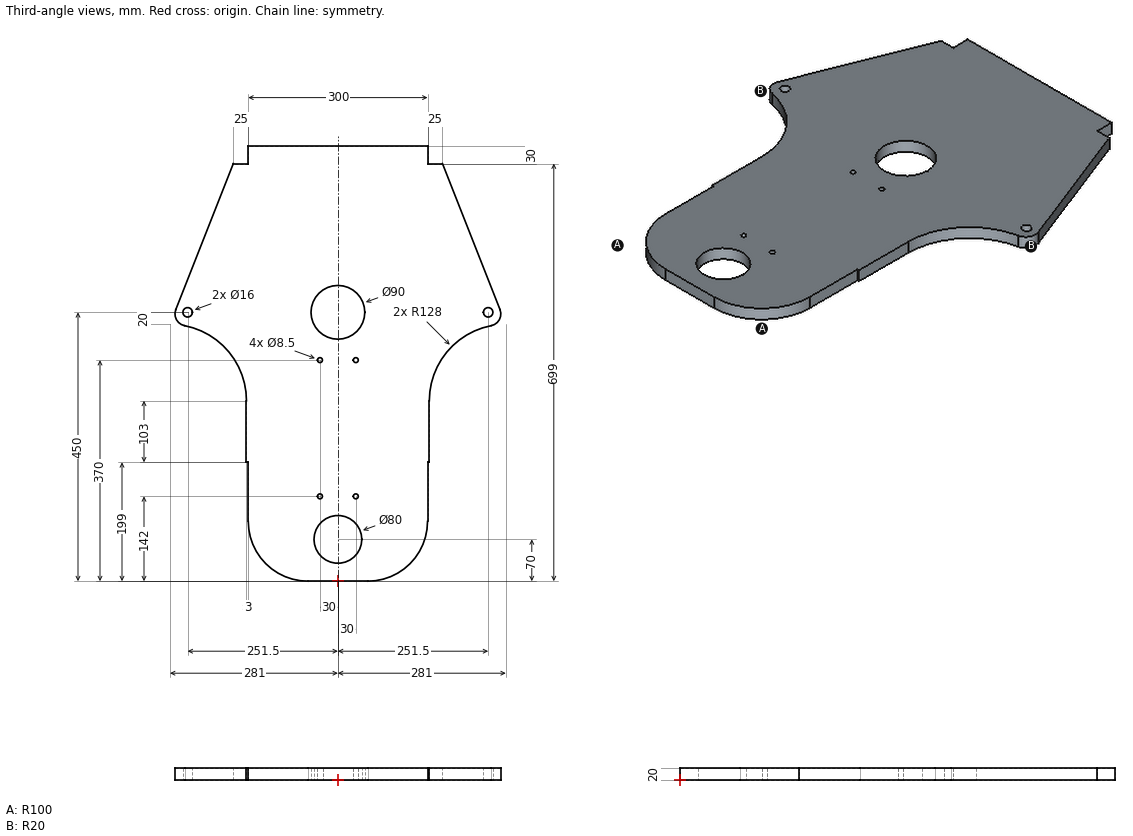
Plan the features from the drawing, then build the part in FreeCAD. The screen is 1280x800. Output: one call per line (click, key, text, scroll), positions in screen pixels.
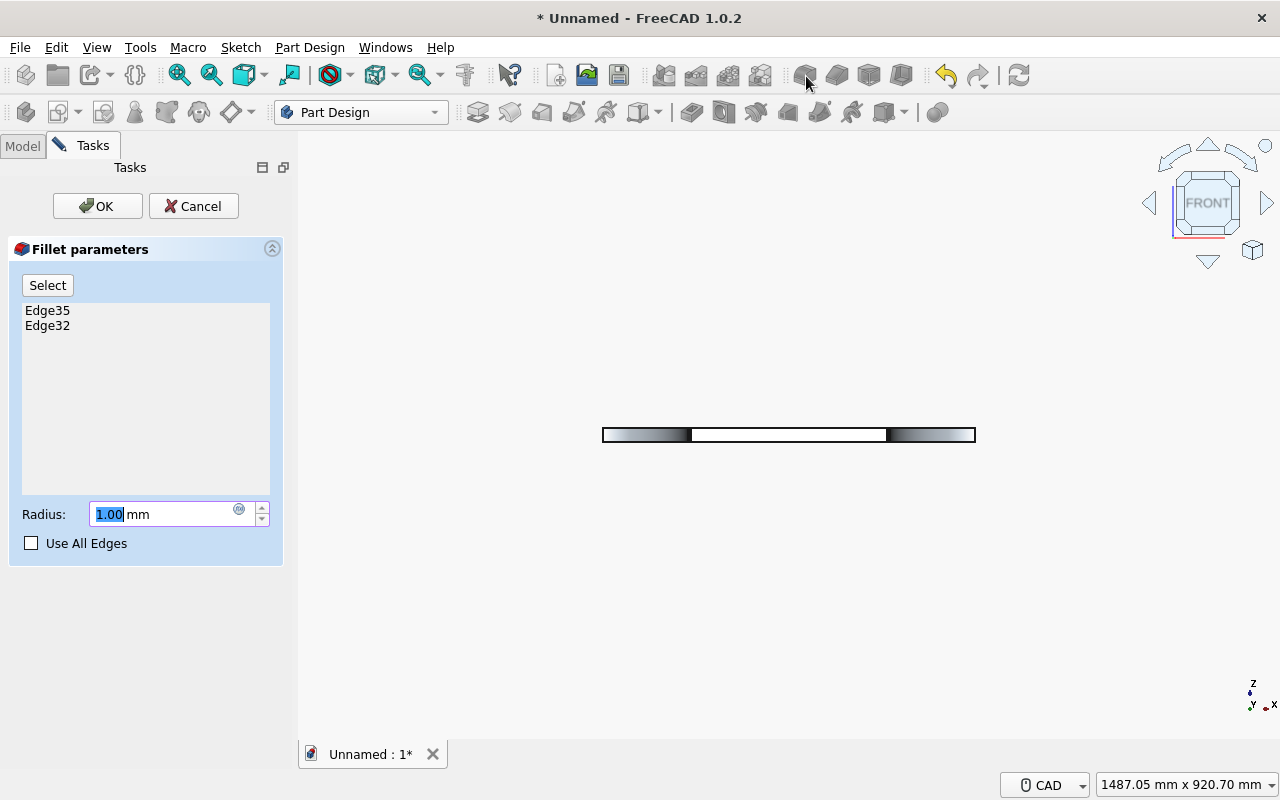
text(100)
key(Tab)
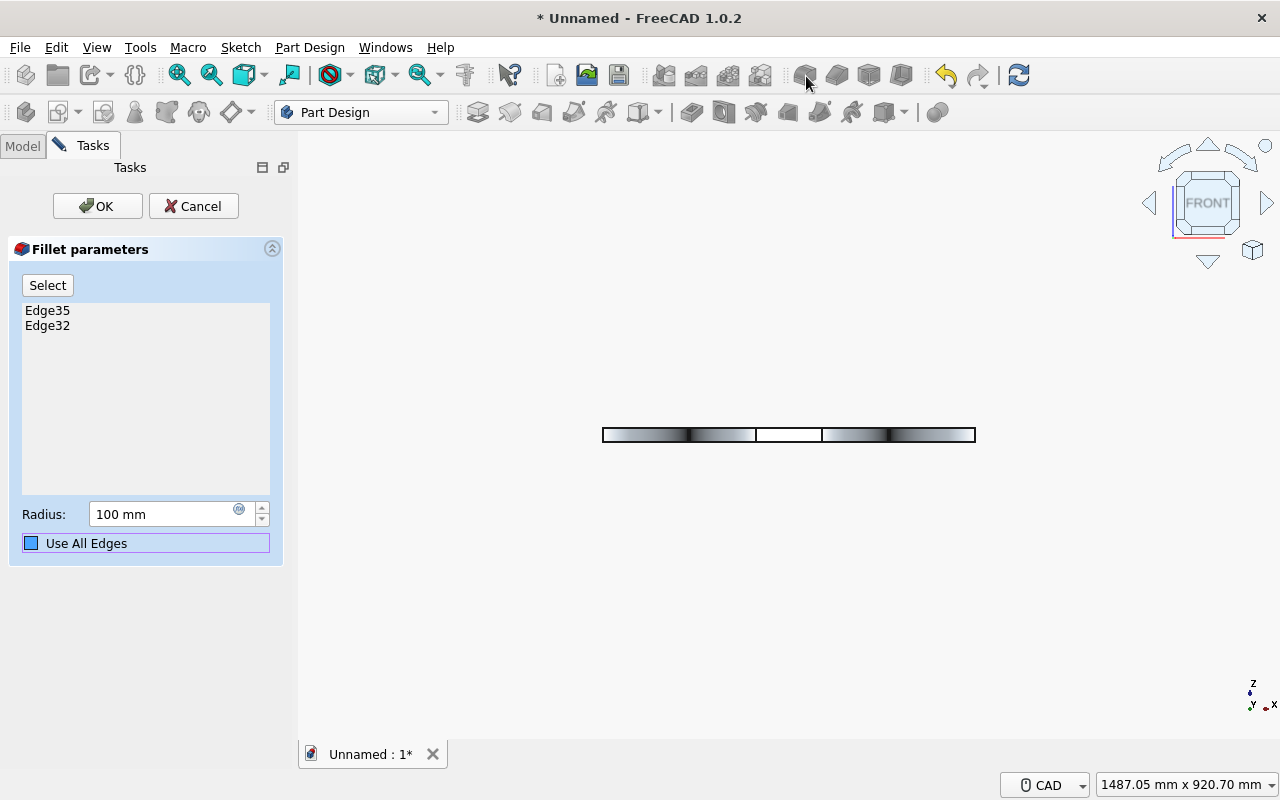
click(98, 206)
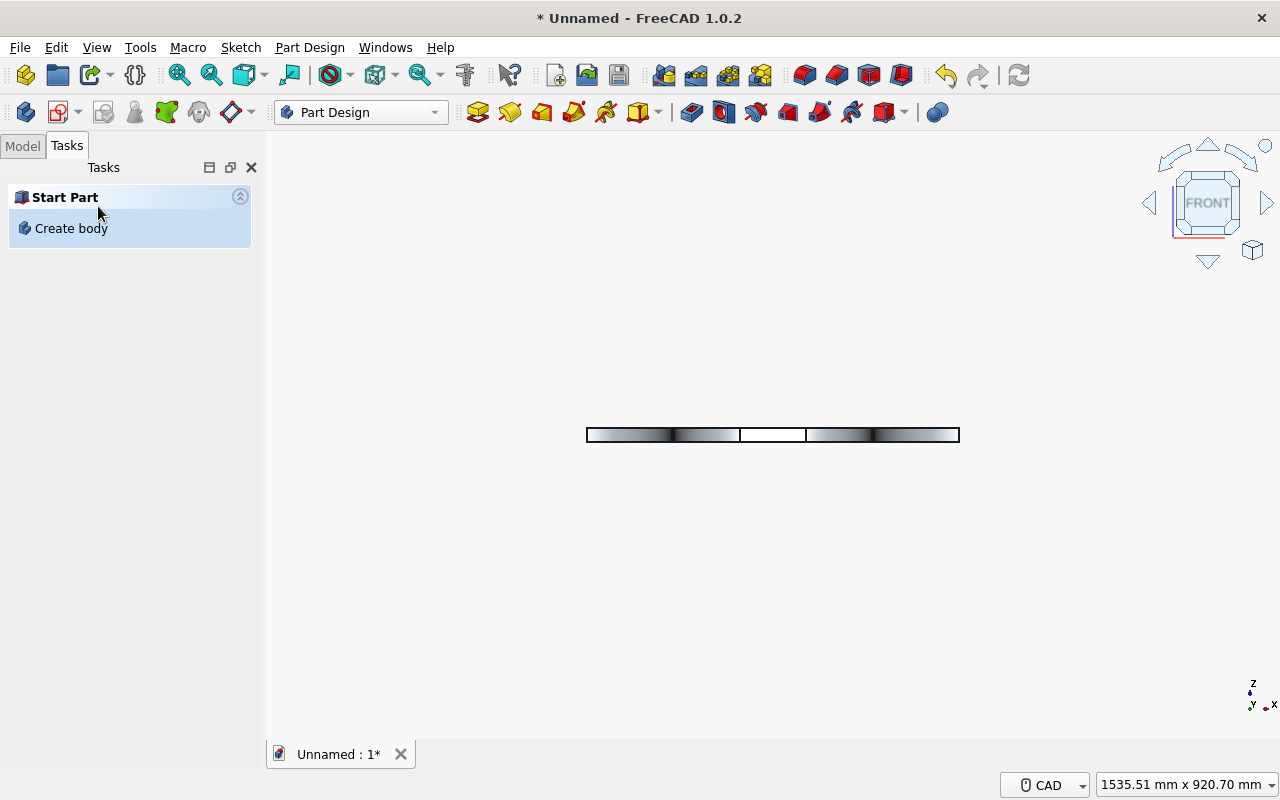
click(180, 76)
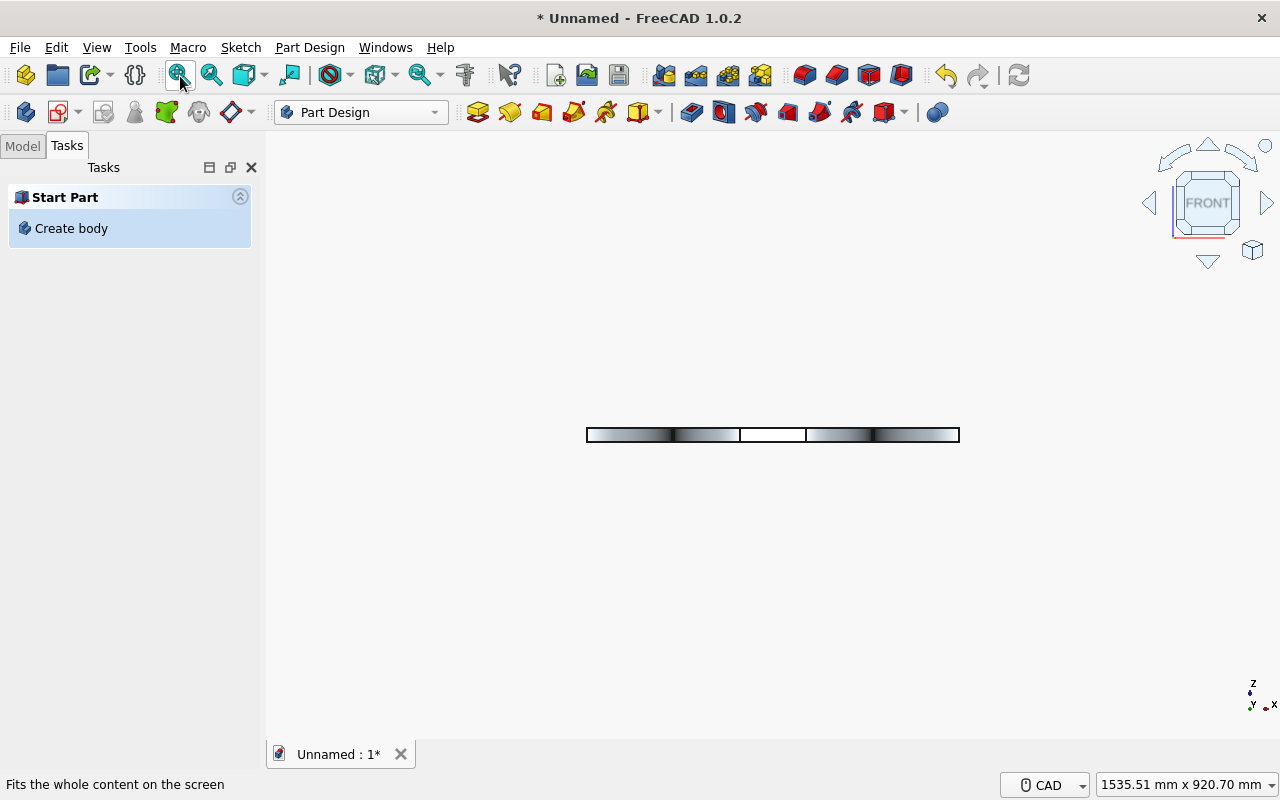
scroll(587, 434, up, 6)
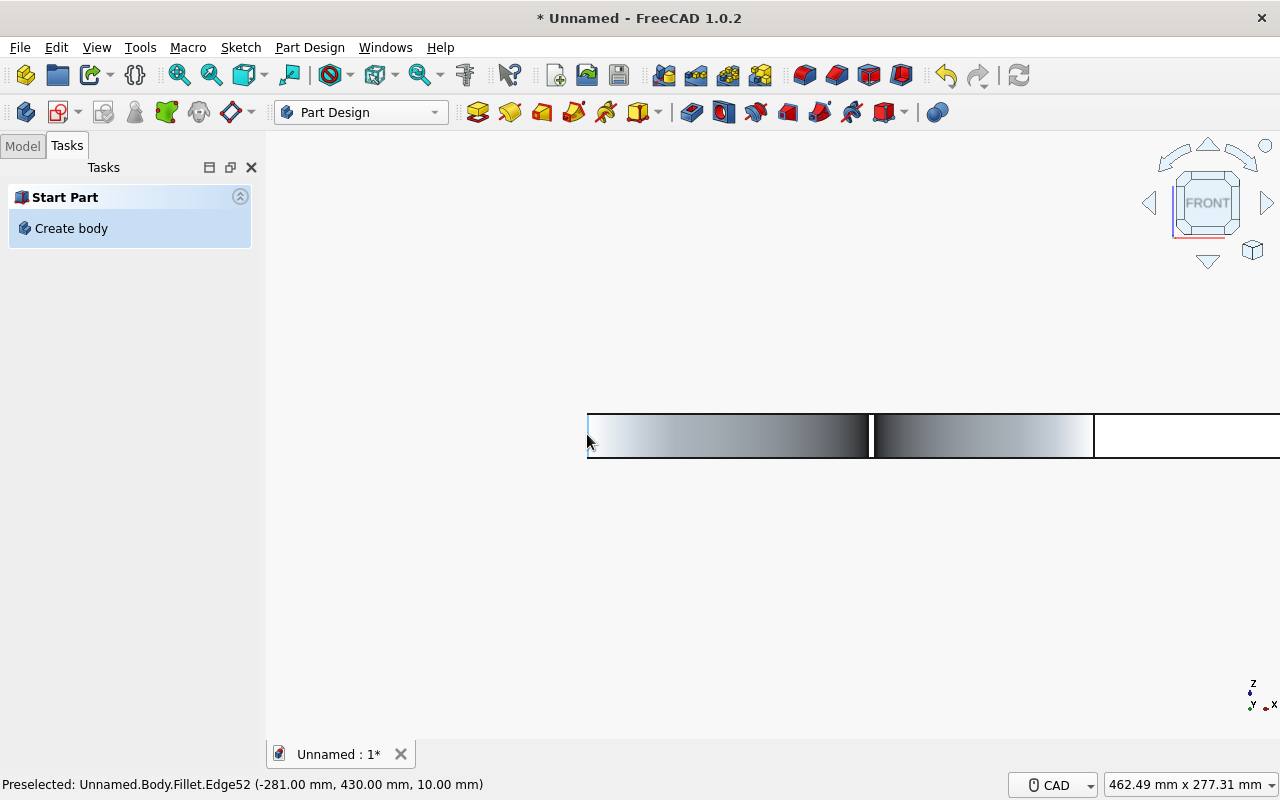
click(180, 76)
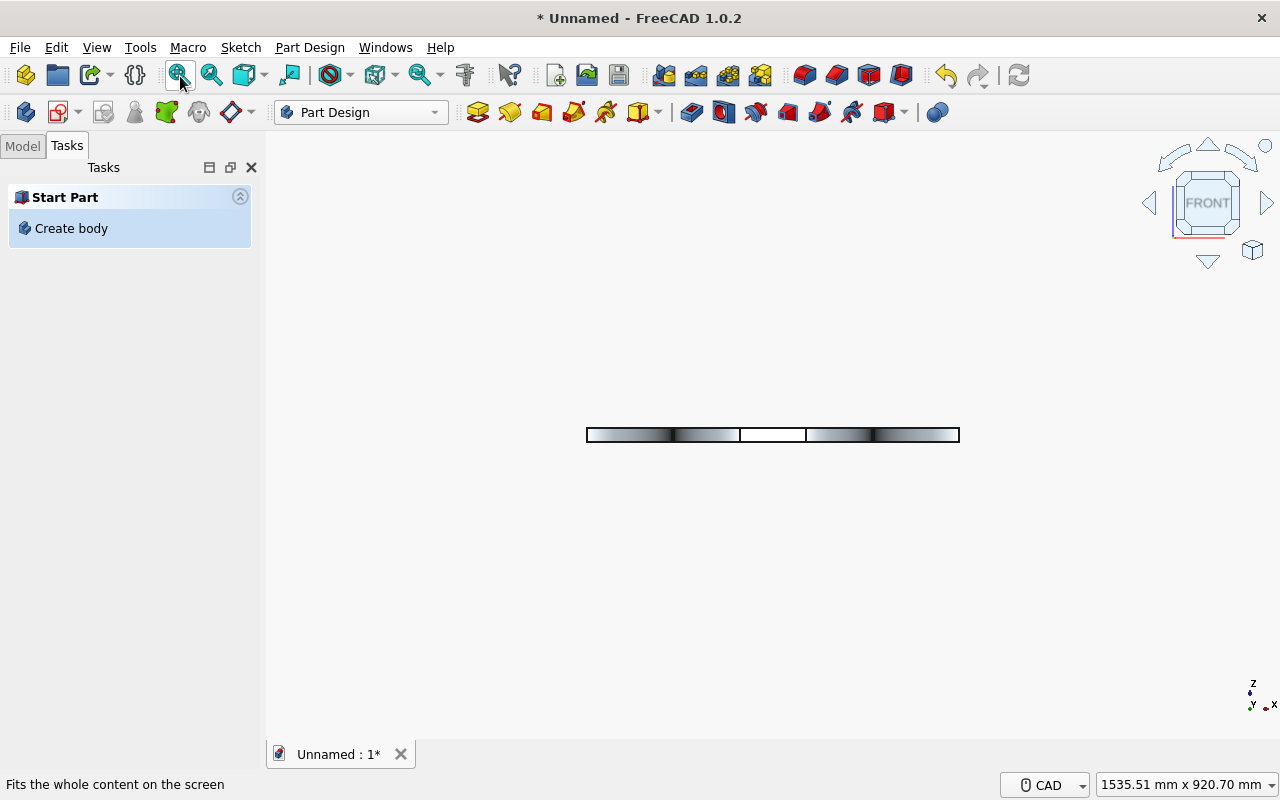
key(0)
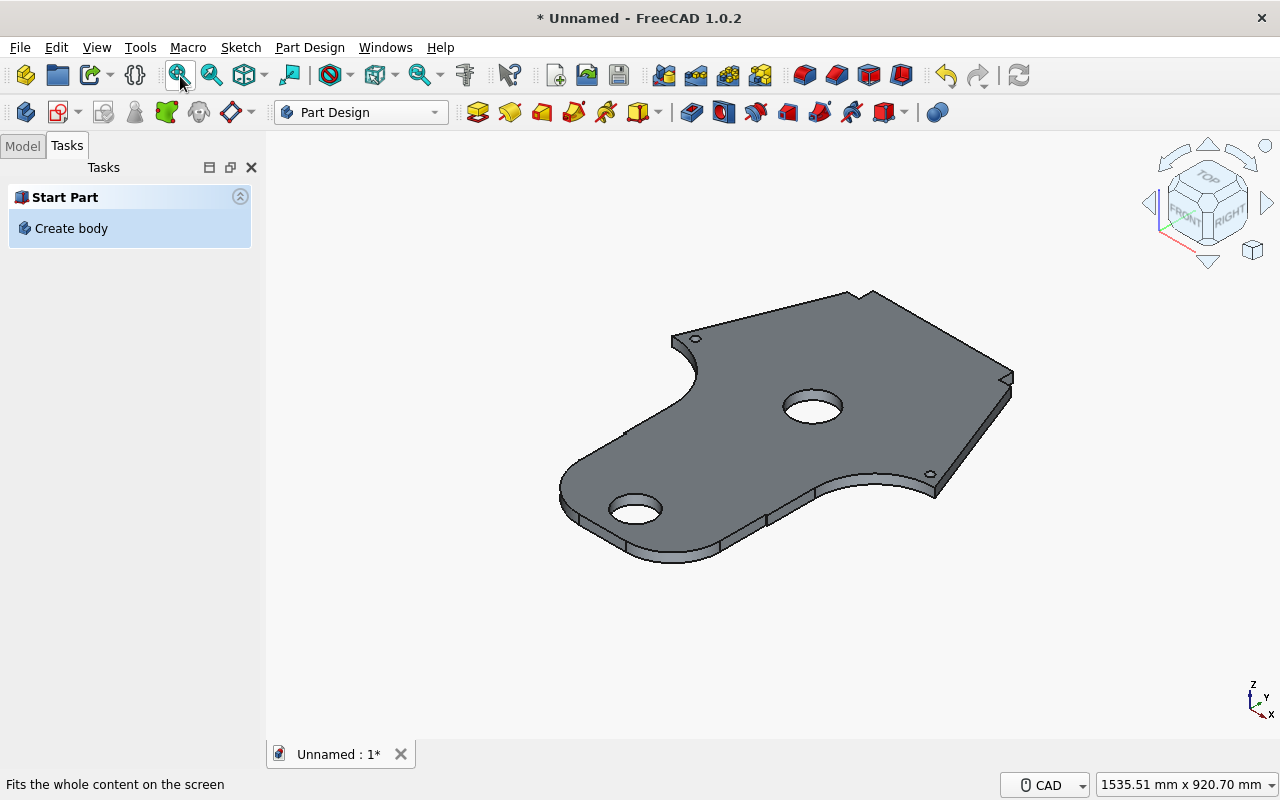
click(935, 493)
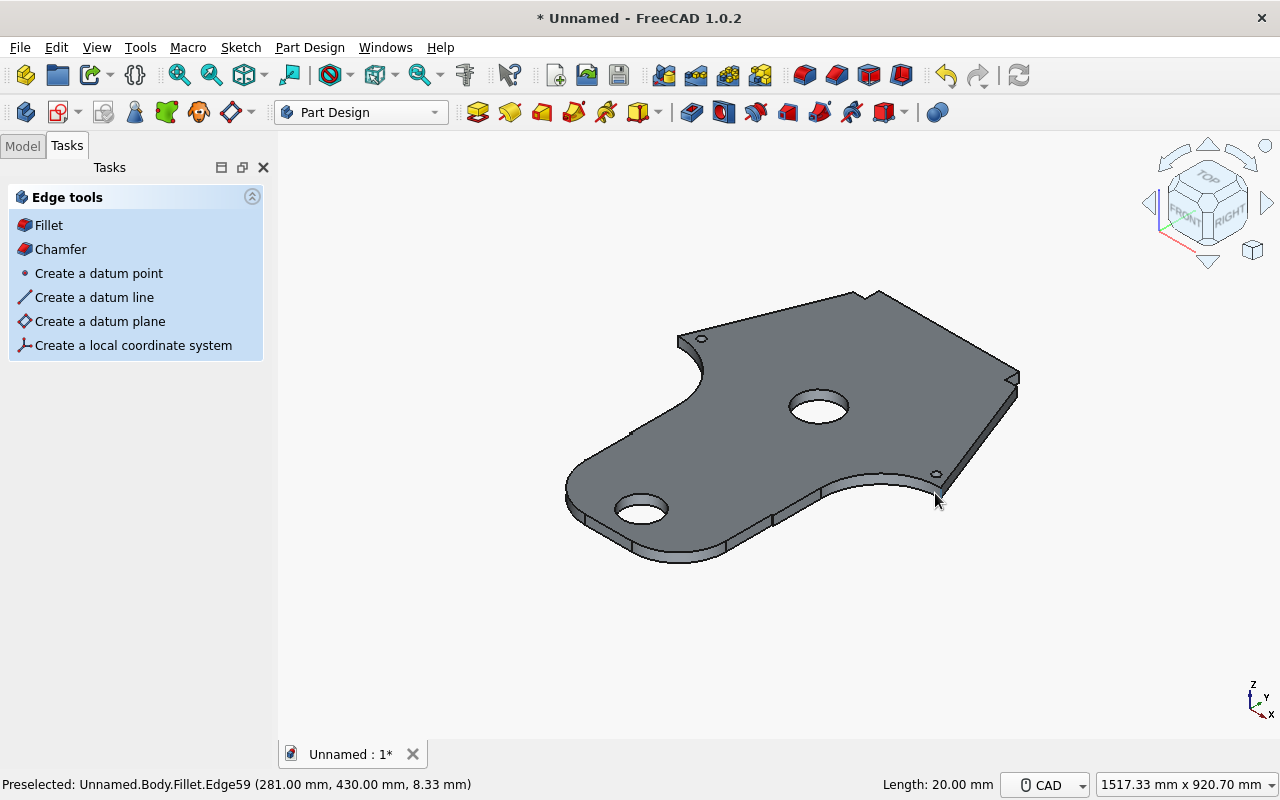
scroll(678, 341, up, 6)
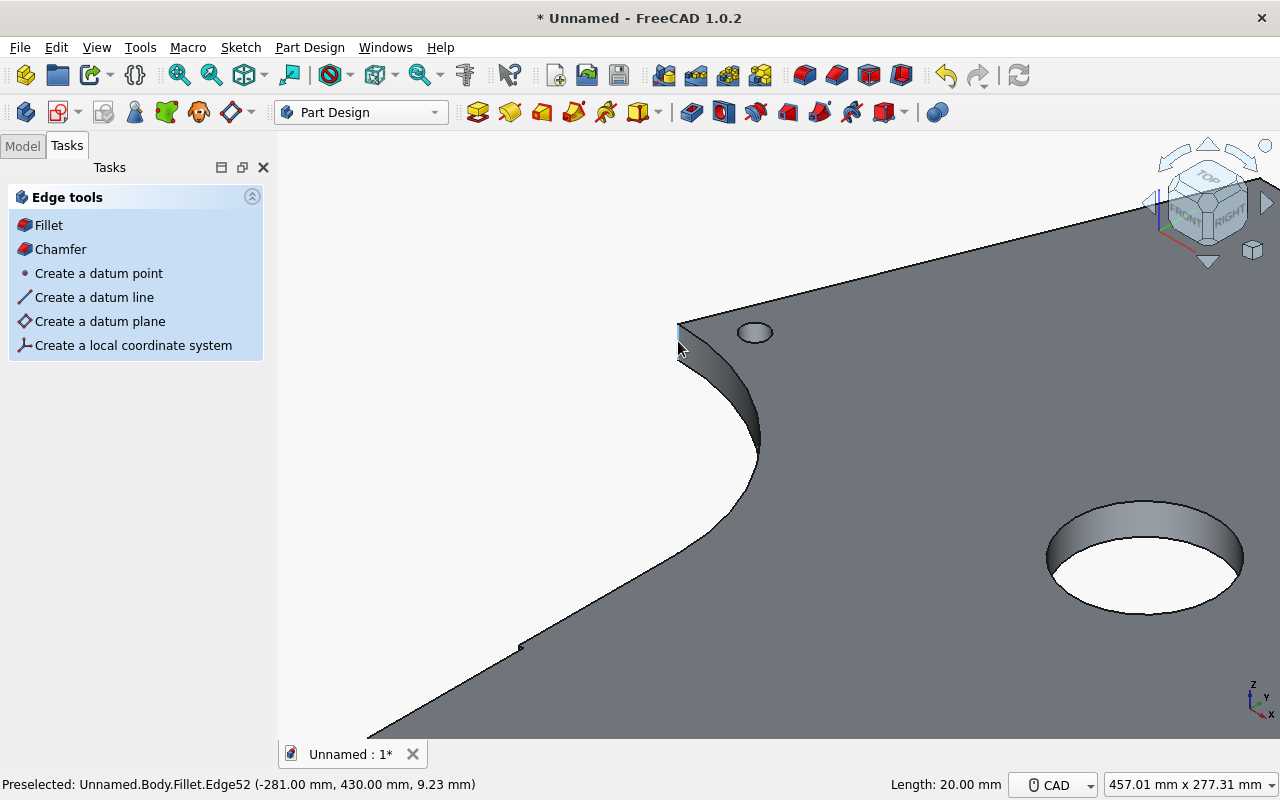
key(v)
key(f)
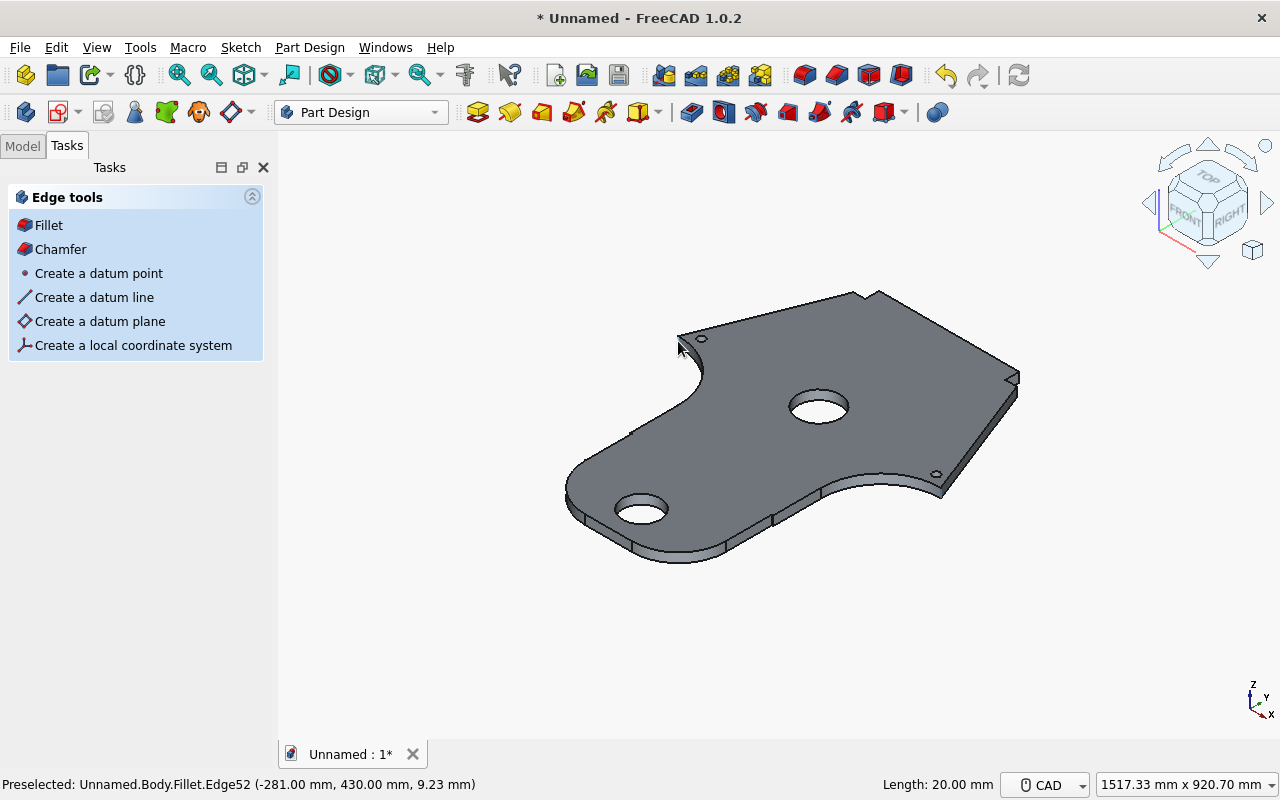
key(2)